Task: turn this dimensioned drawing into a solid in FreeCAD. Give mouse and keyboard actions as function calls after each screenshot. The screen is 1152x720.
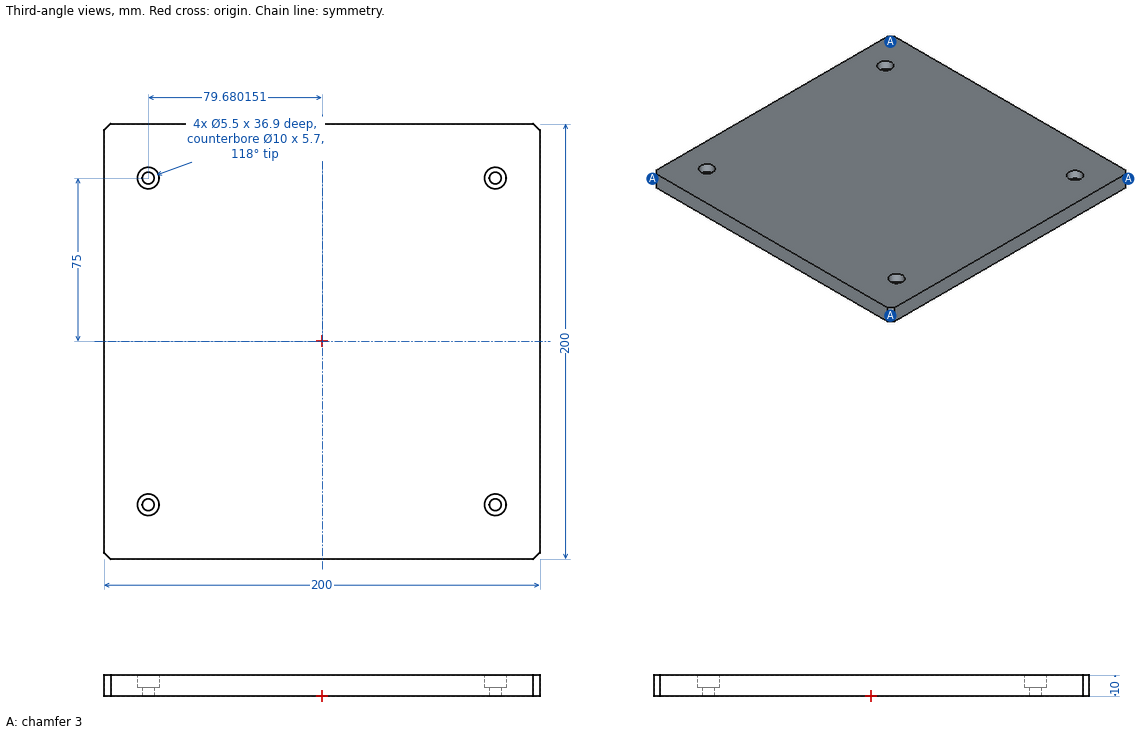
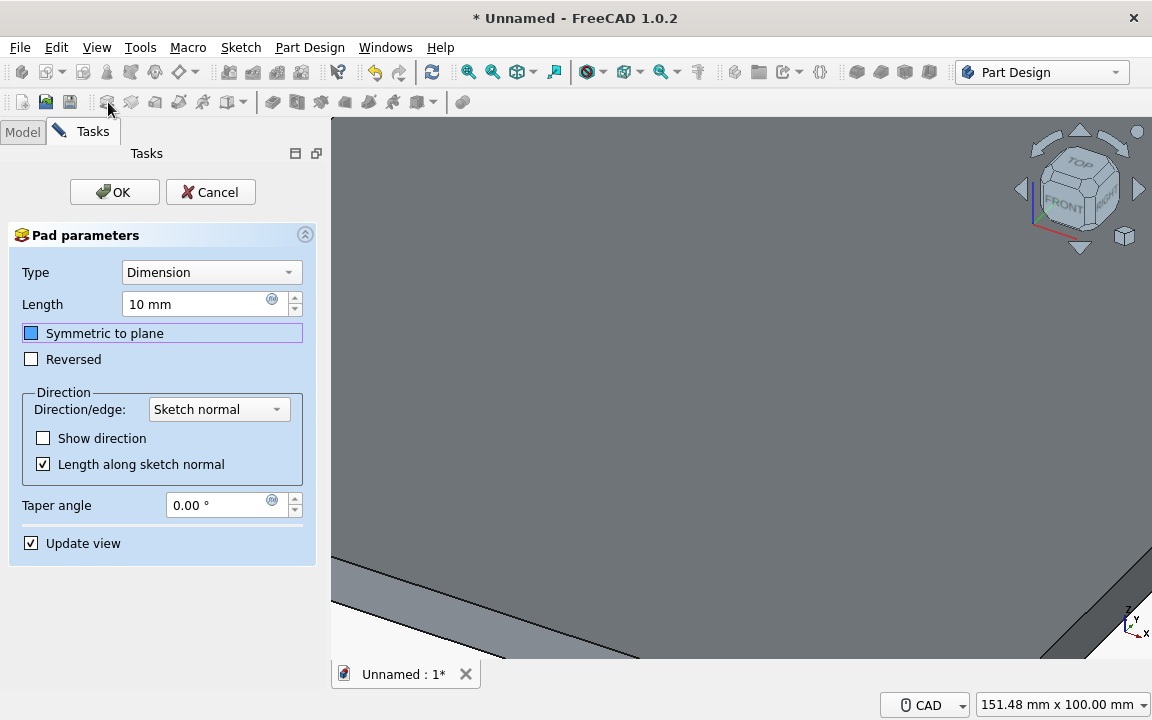
click(115, 192)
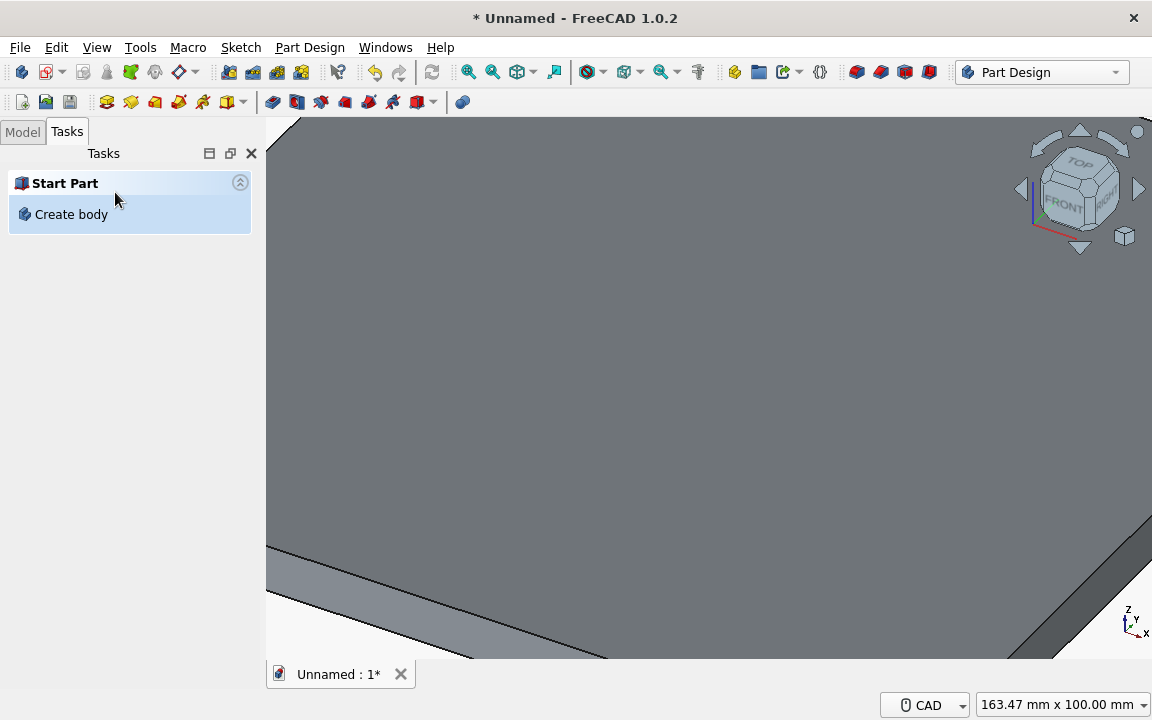
click(470, 72)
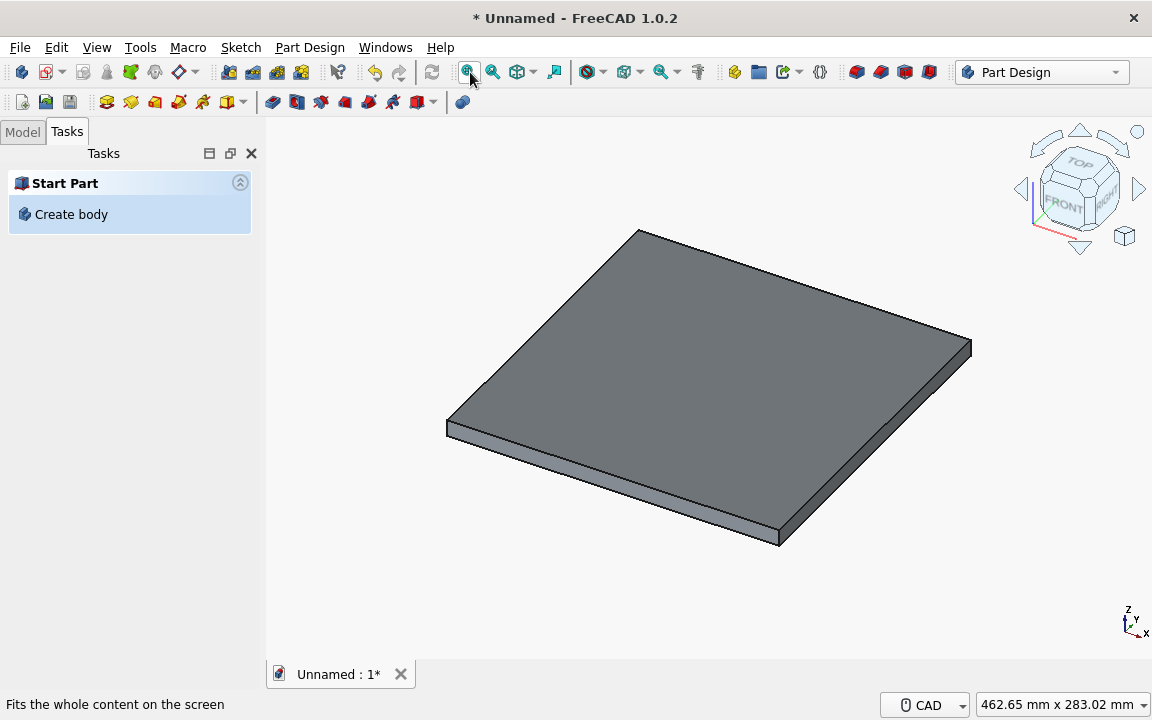
click(709, 379)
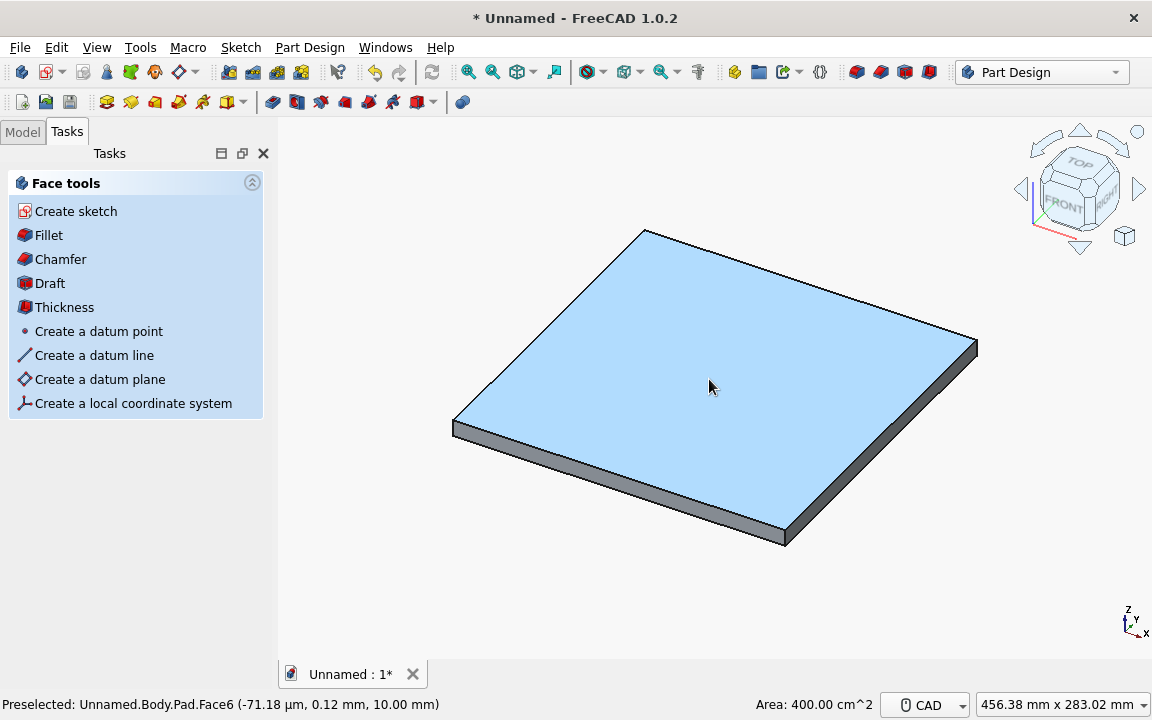
click(46, 72)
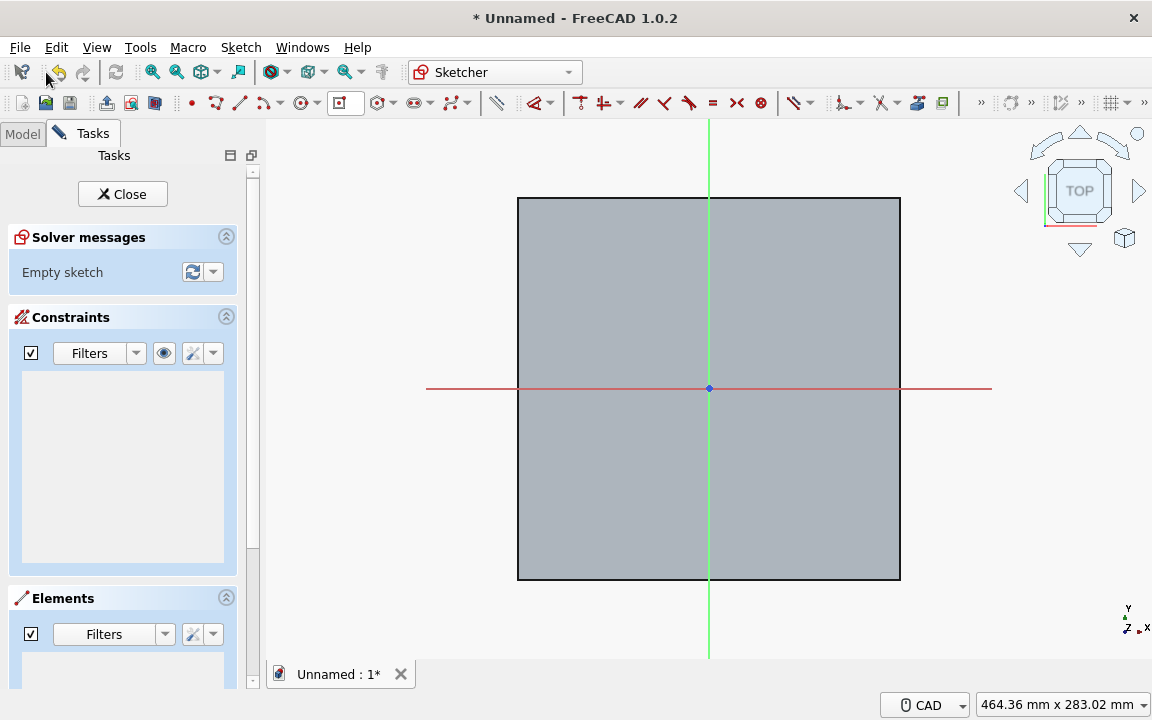
click(302, 104)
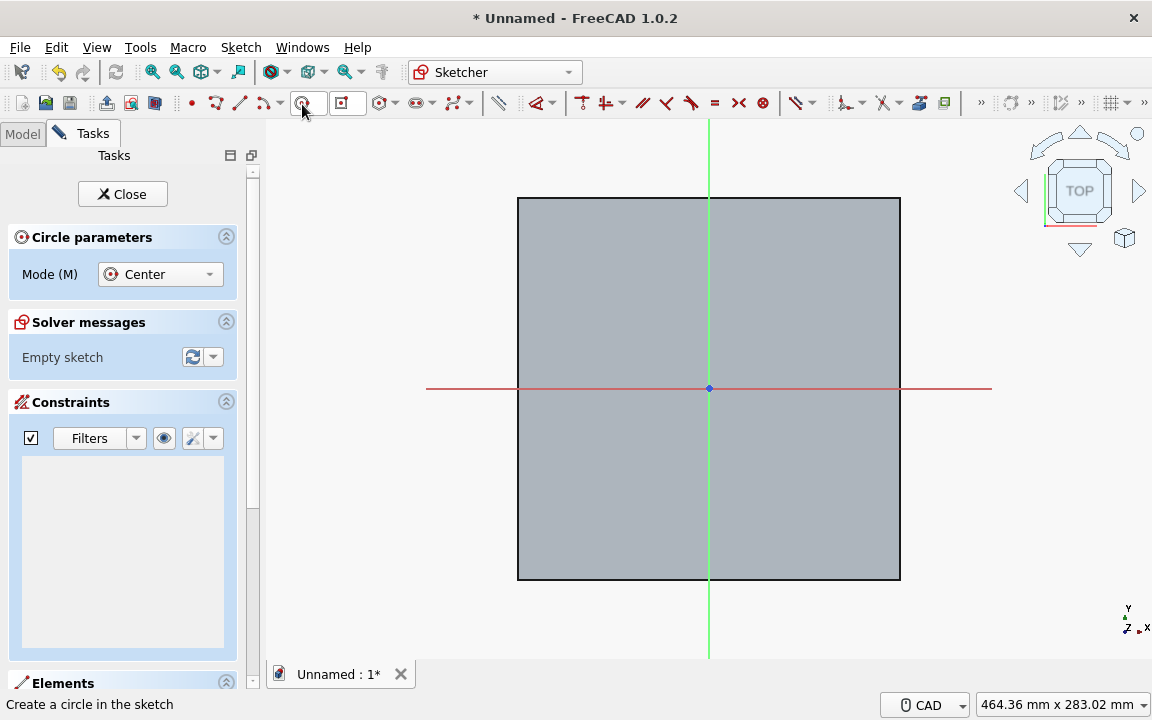
scroll(557, 246, up, 8)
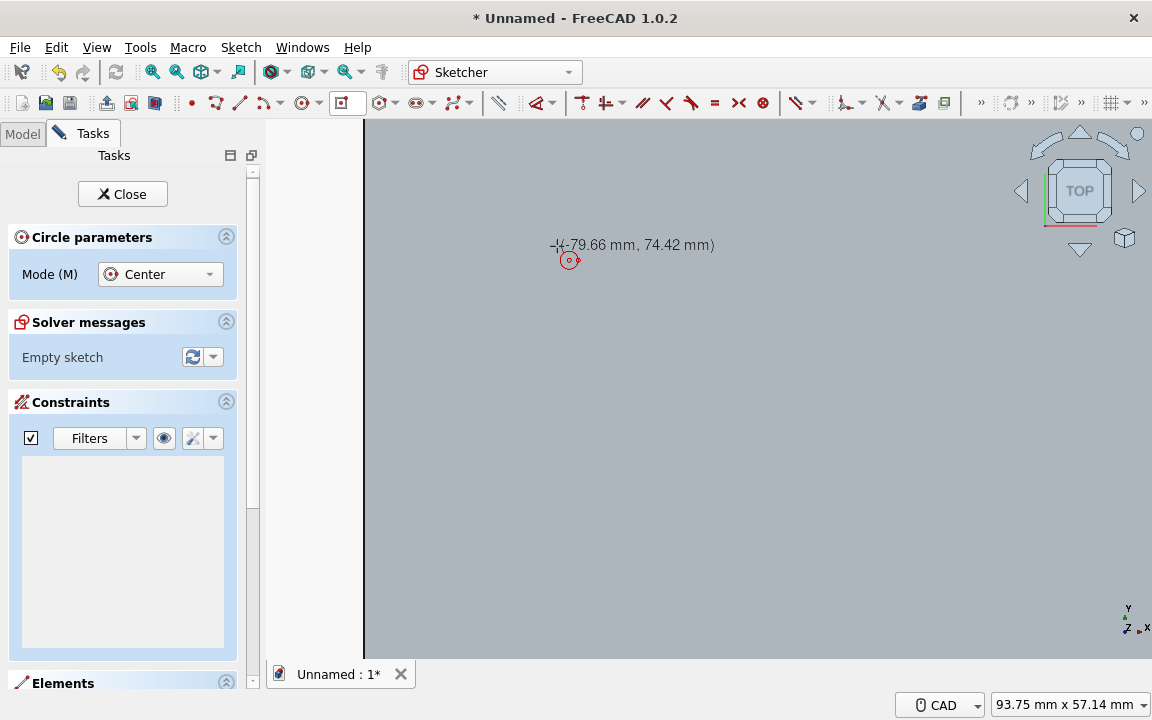
scroll(422, 204, down, 7)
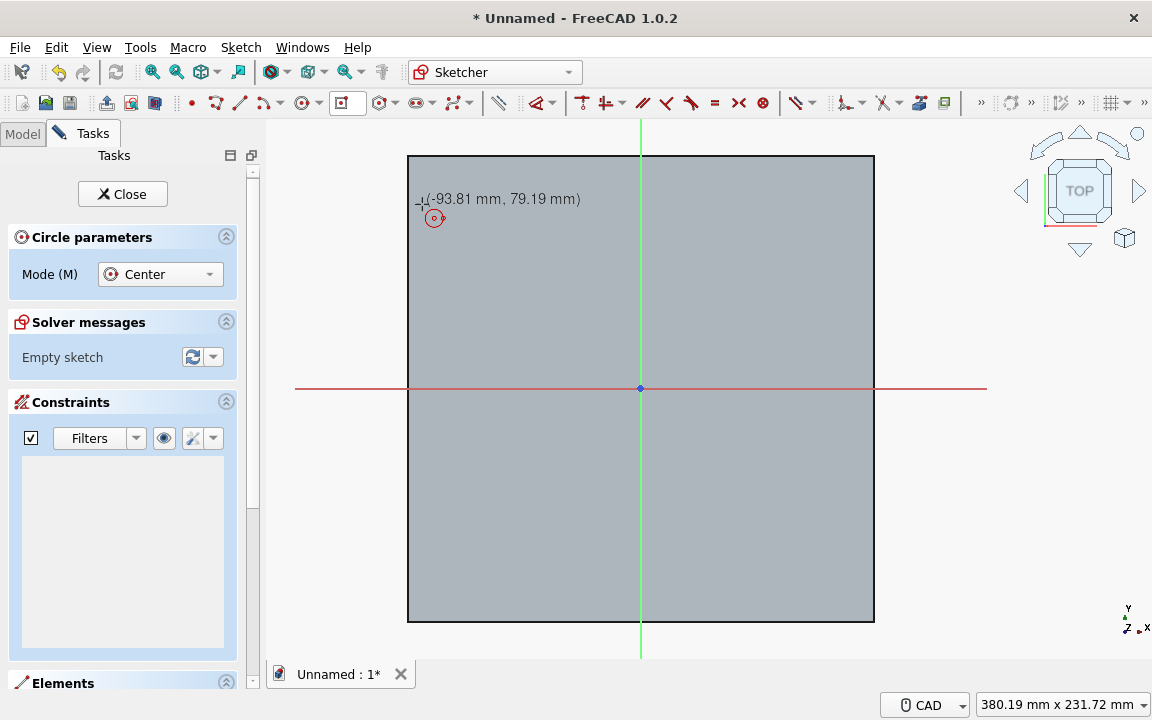
click(455, 214)
move(460, 210)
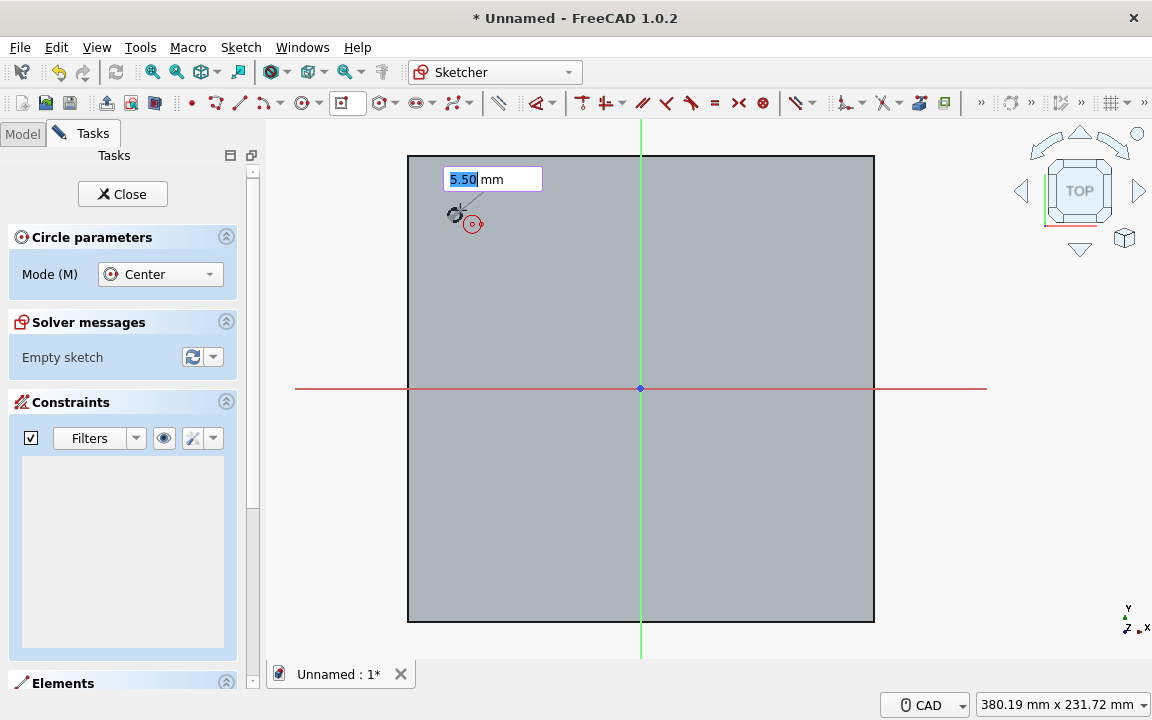
text(5.5)
key(Return)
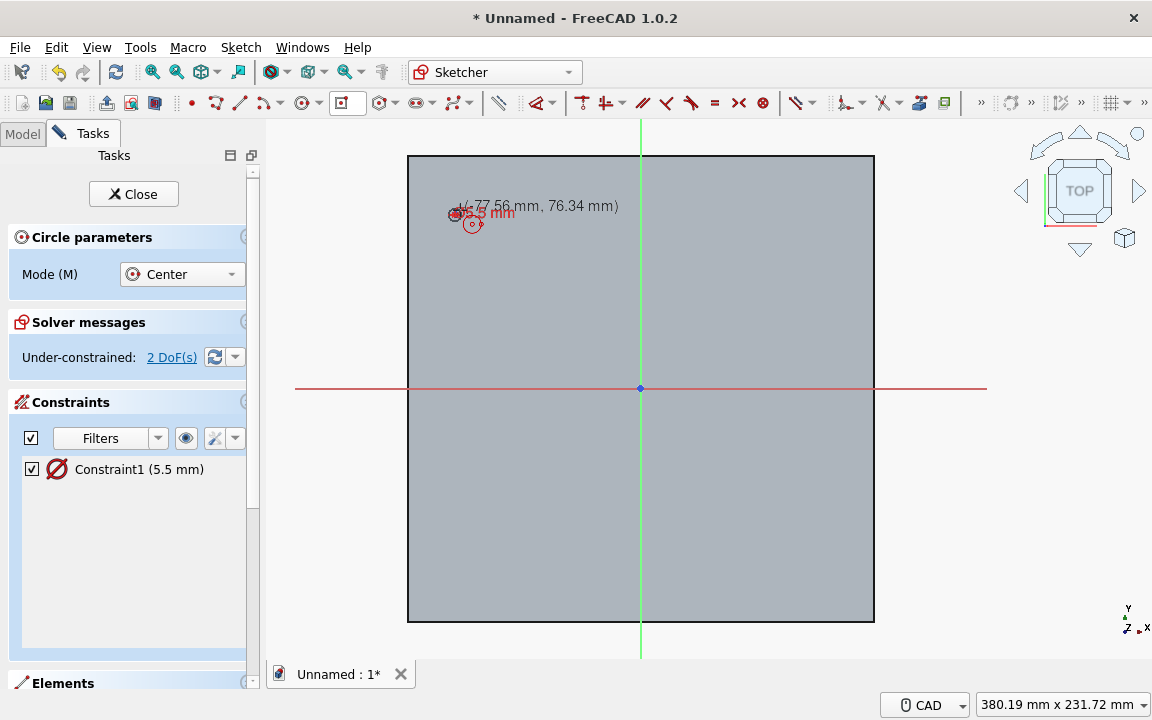
scroll(826, 214, up, 7)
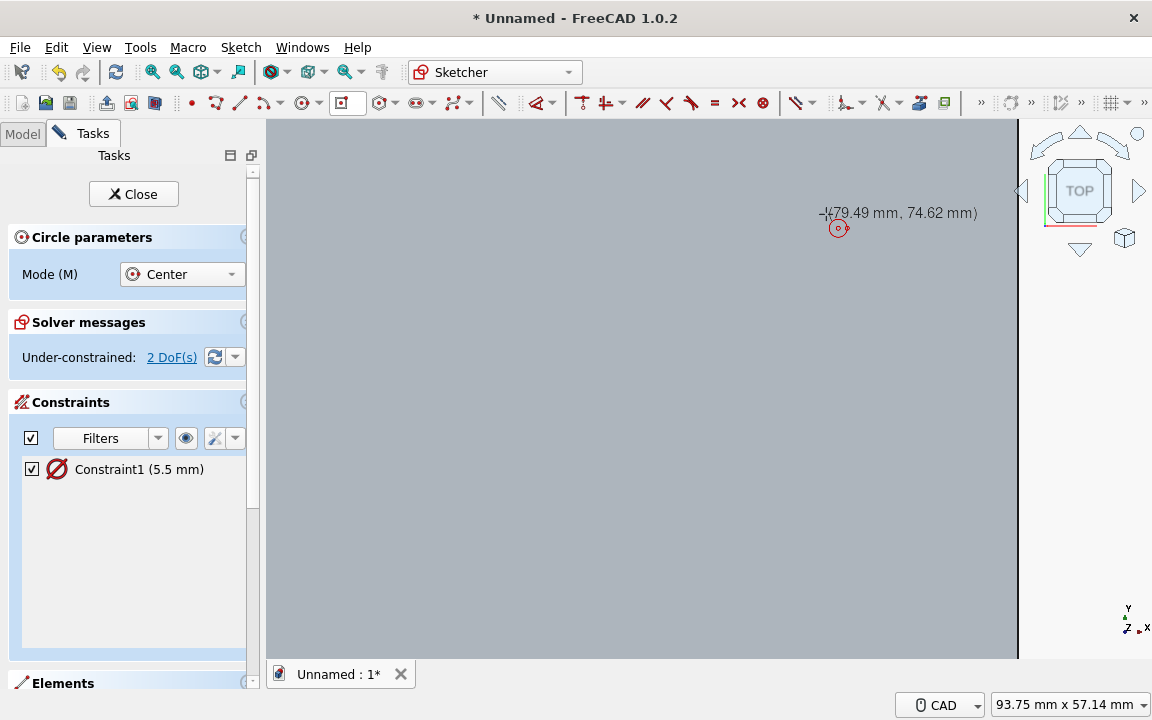
scroll(826, 214, down, 7)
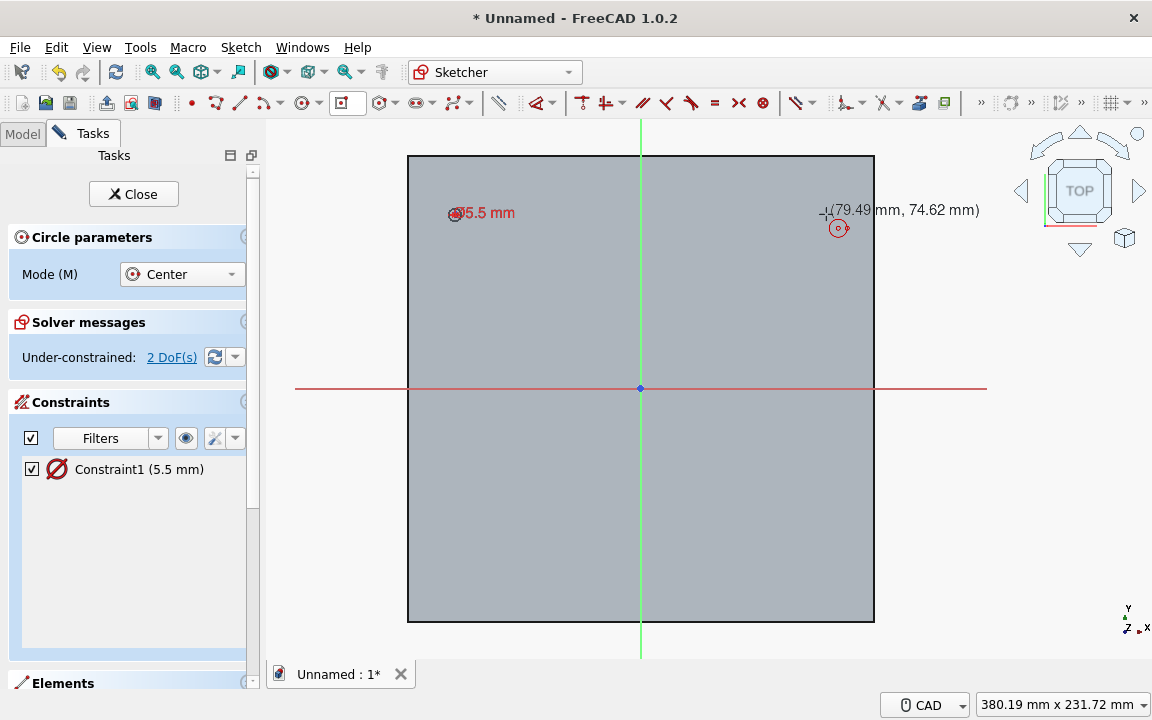
click(826, 214)
move(831, 210)